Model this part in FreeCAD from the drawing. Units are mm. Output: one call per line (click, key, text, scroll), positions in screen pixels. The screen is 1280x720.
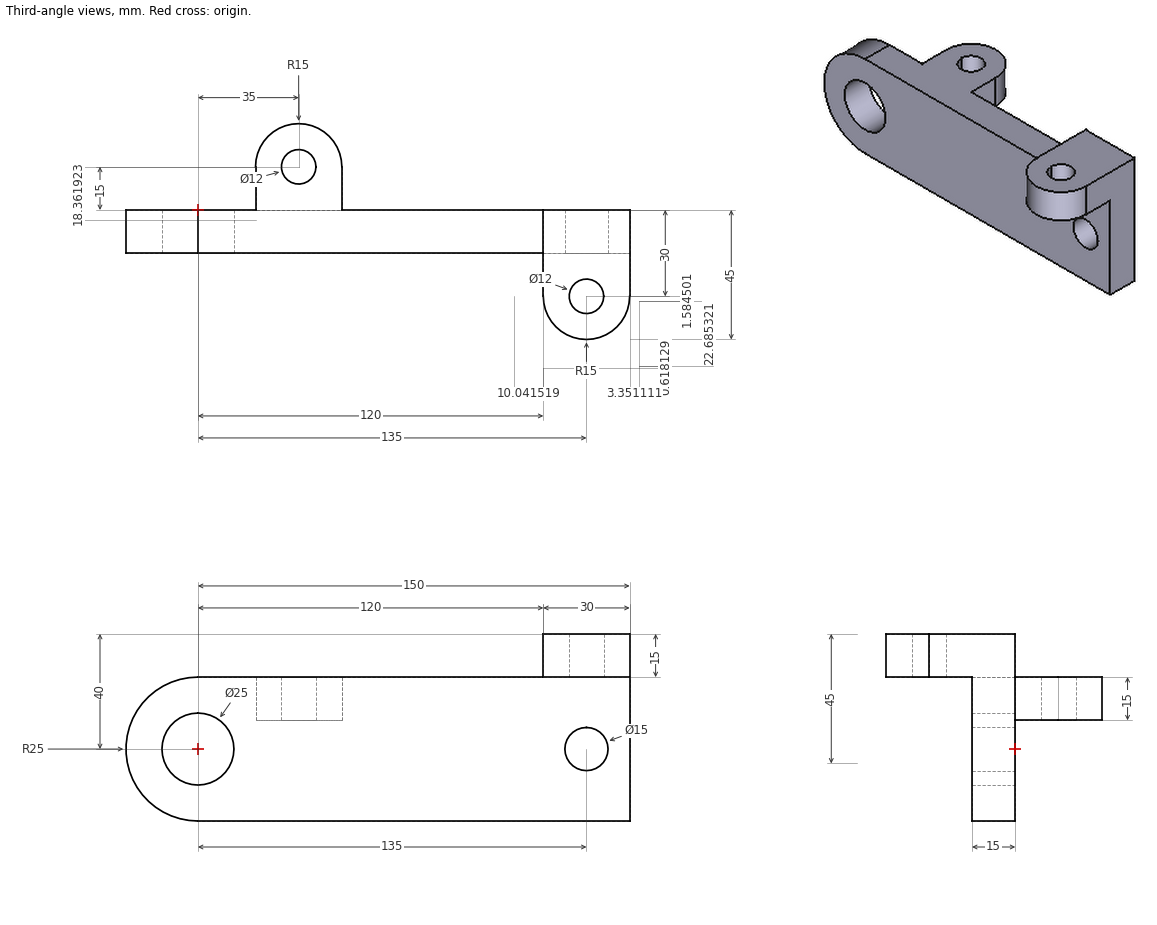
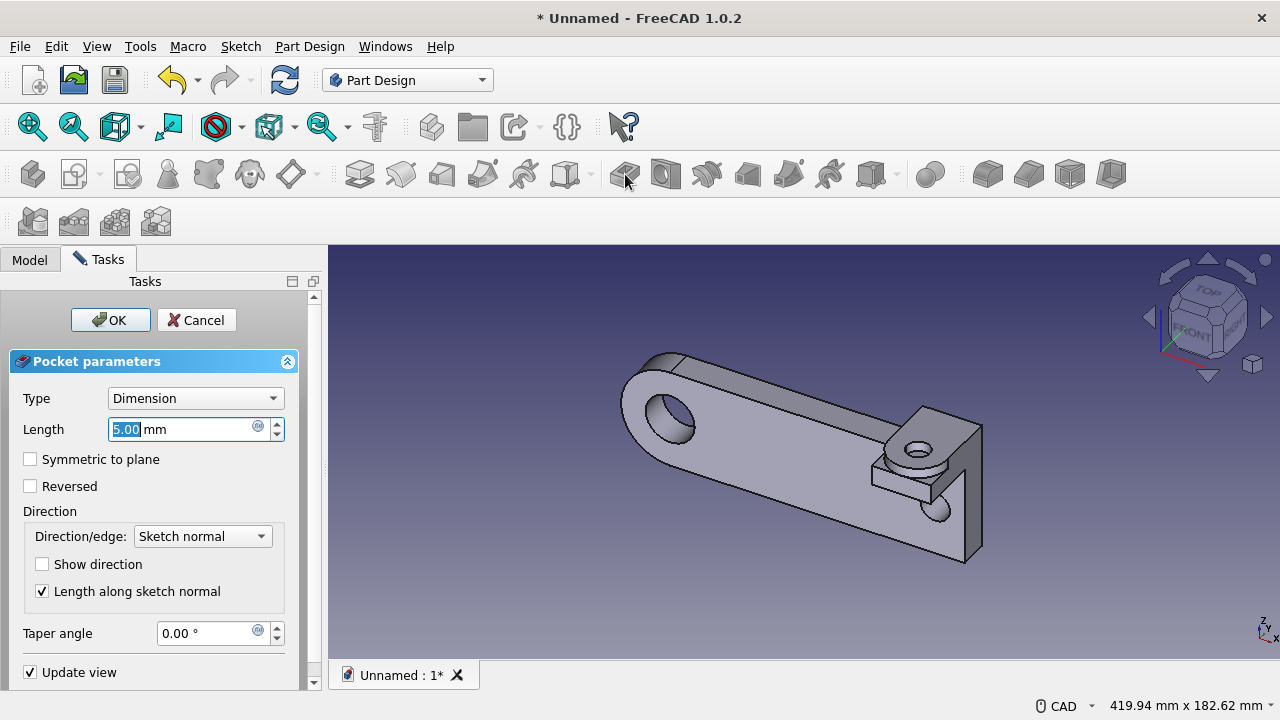
text(45)
key(Tab)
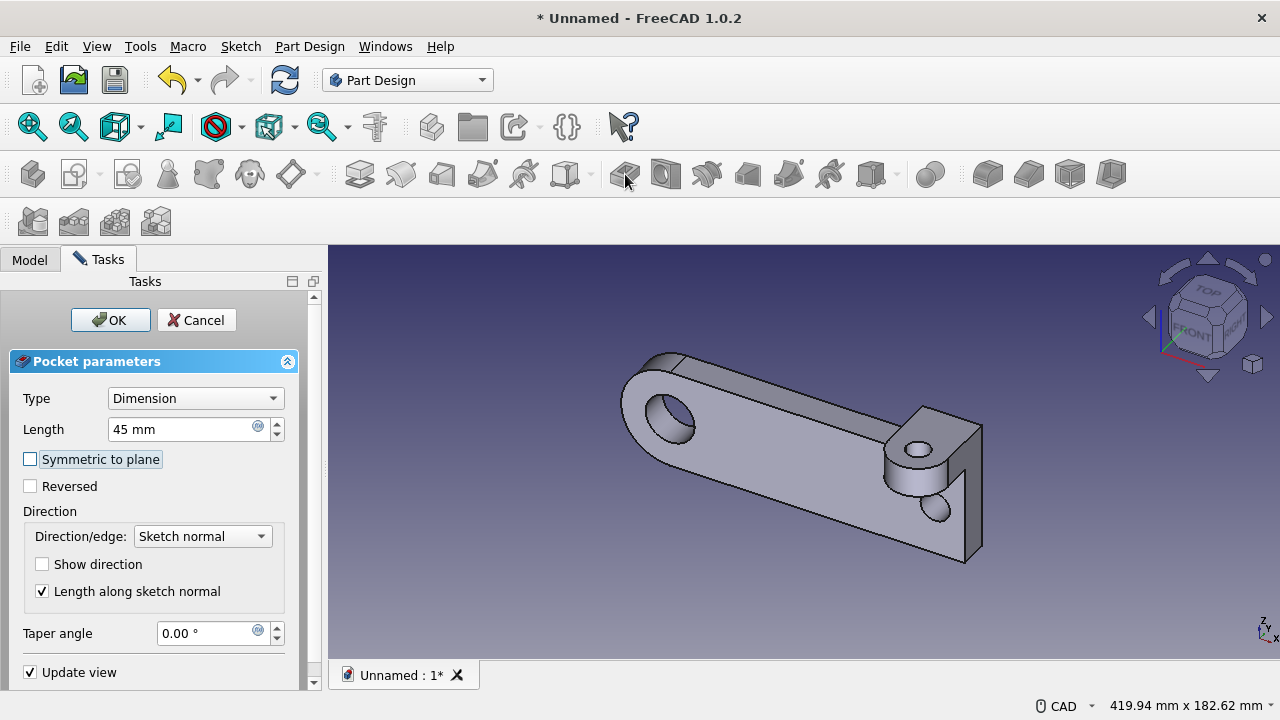
click(111, 320)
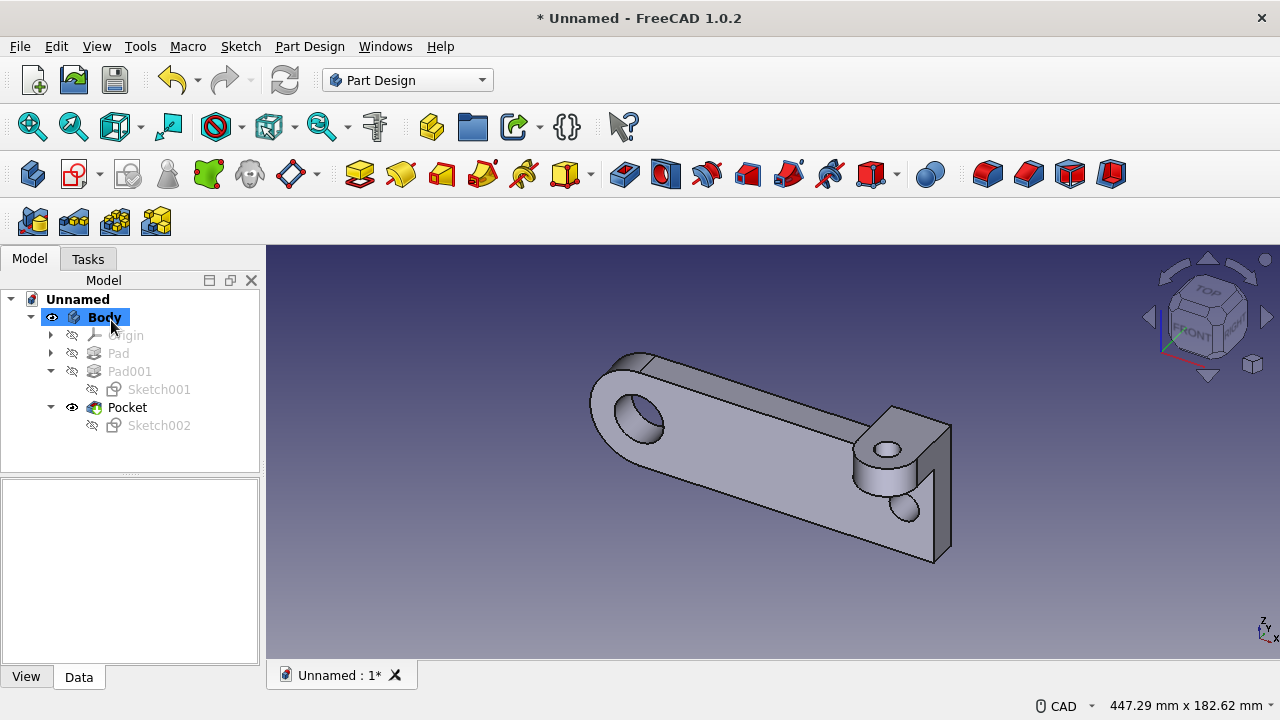
click(833, 425)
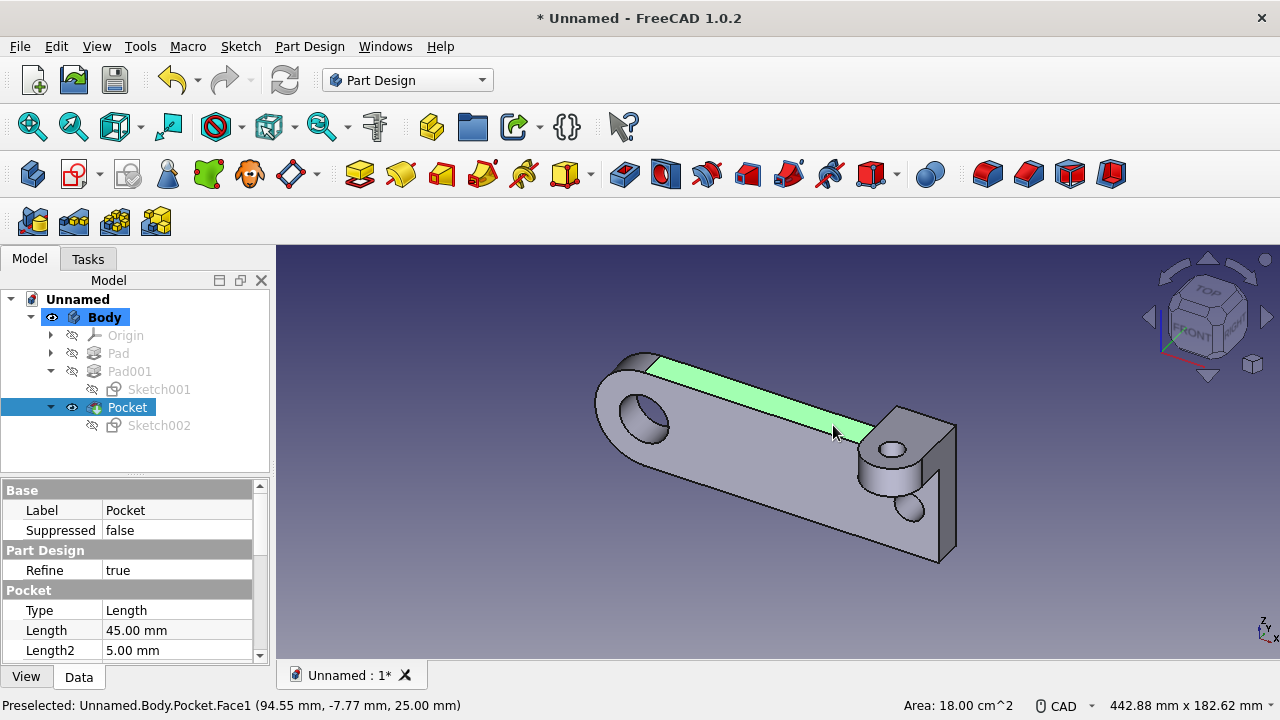
click(74, 174)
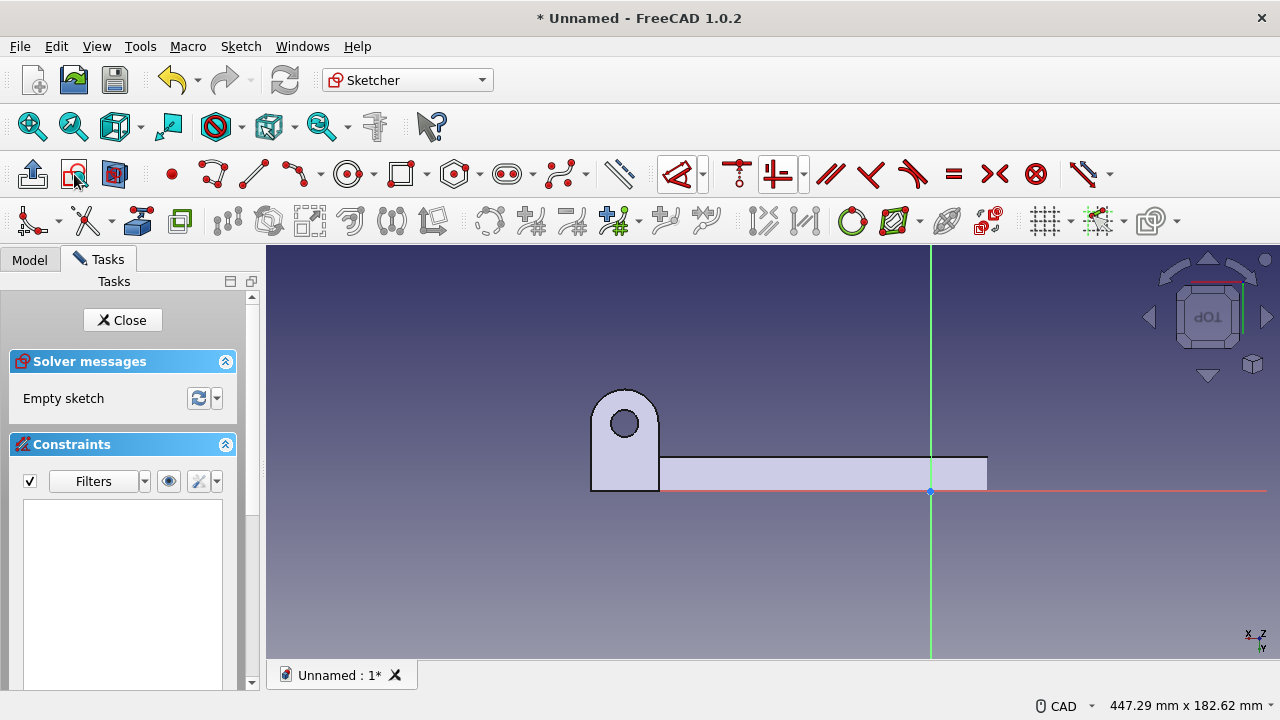
click(115, 174)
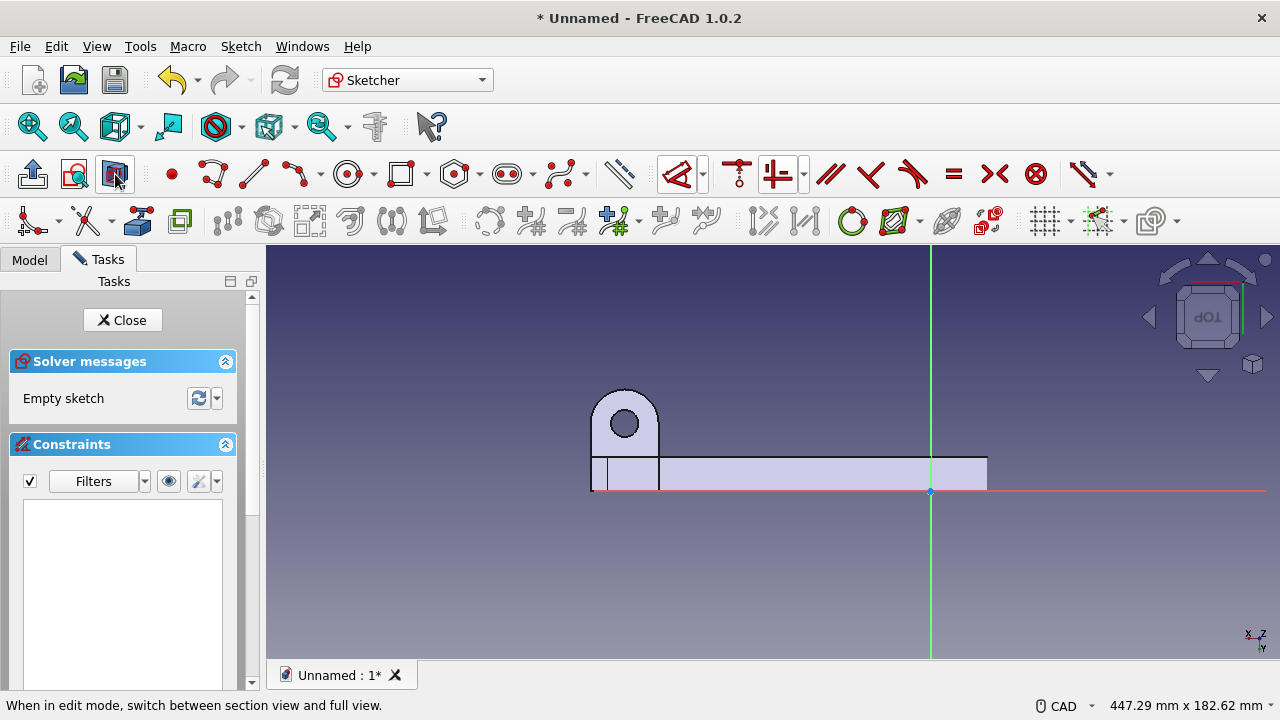
scroll(947, 552, up, 6)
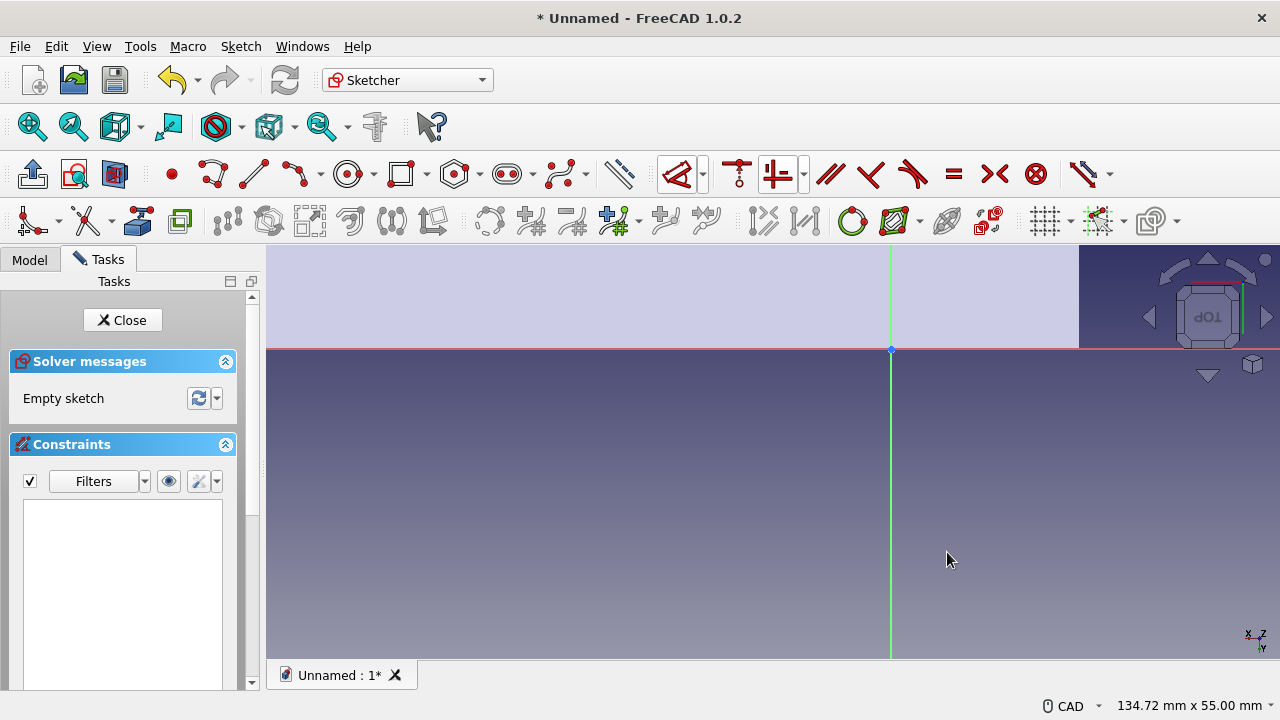
click(213, 174)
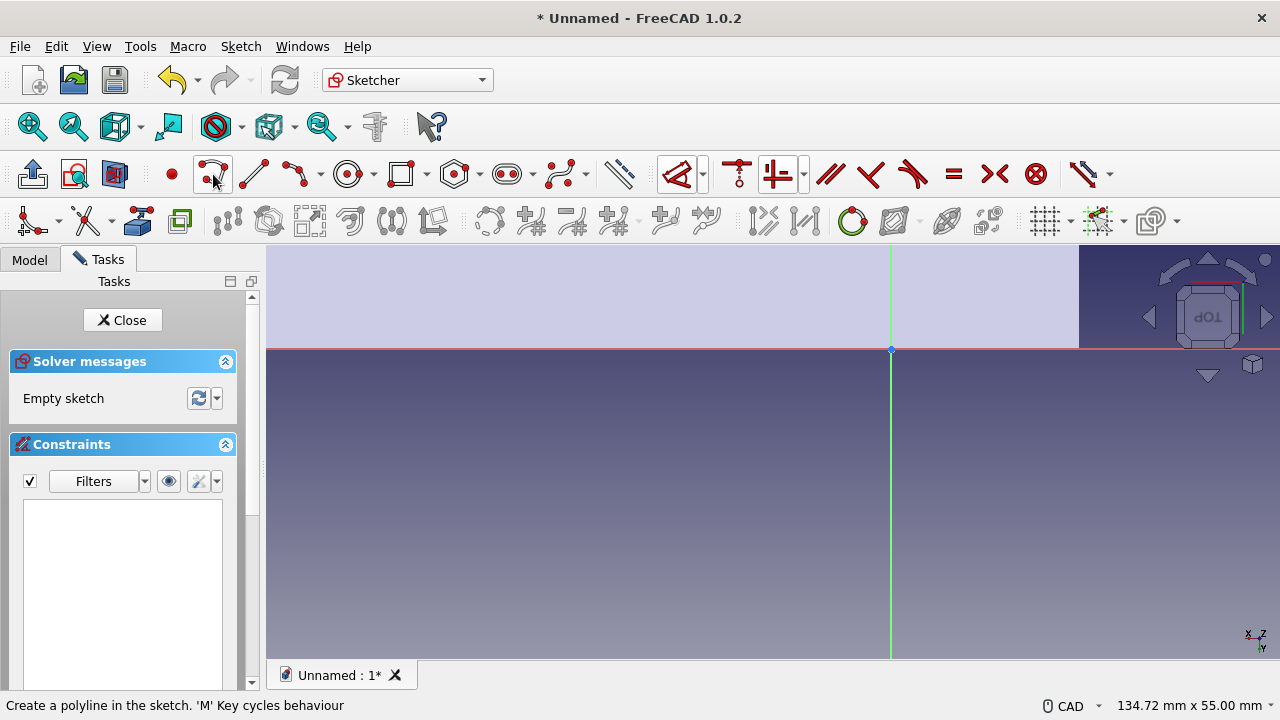
click(741, 462)
click(741, 324)
click(515, 324)
click(515, 462)
right_click(515, 462)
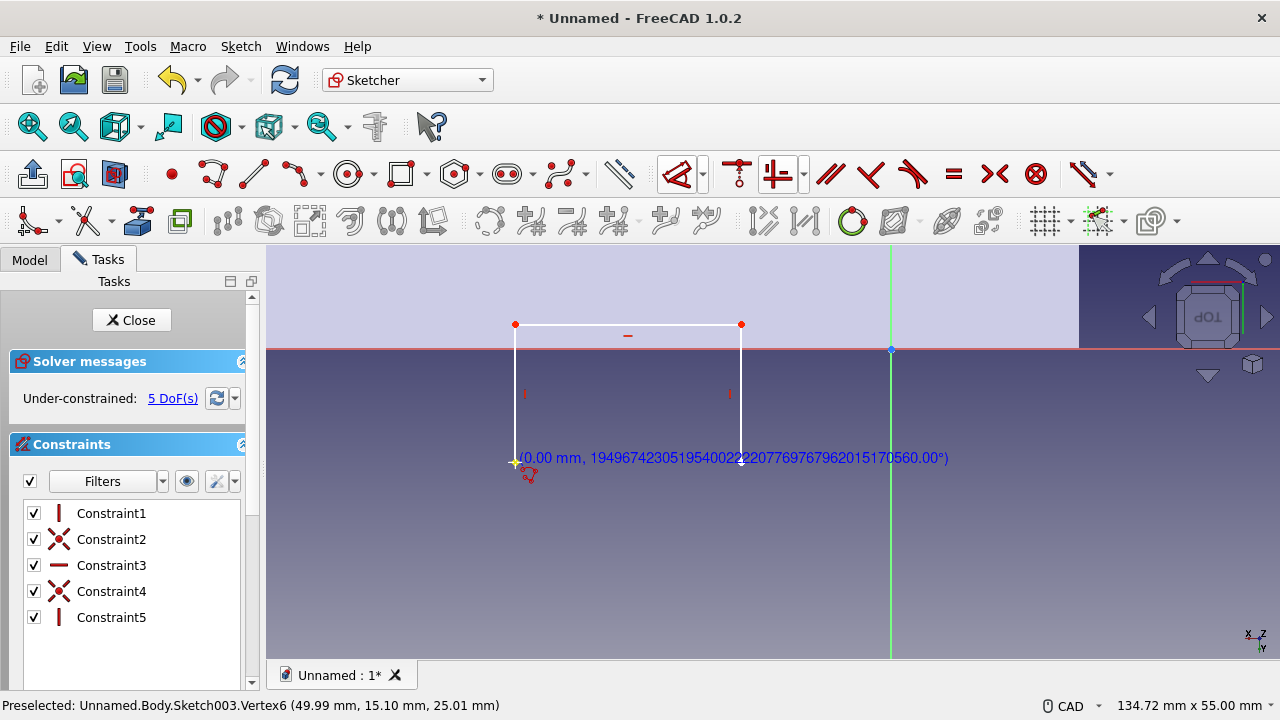
click(294, 174)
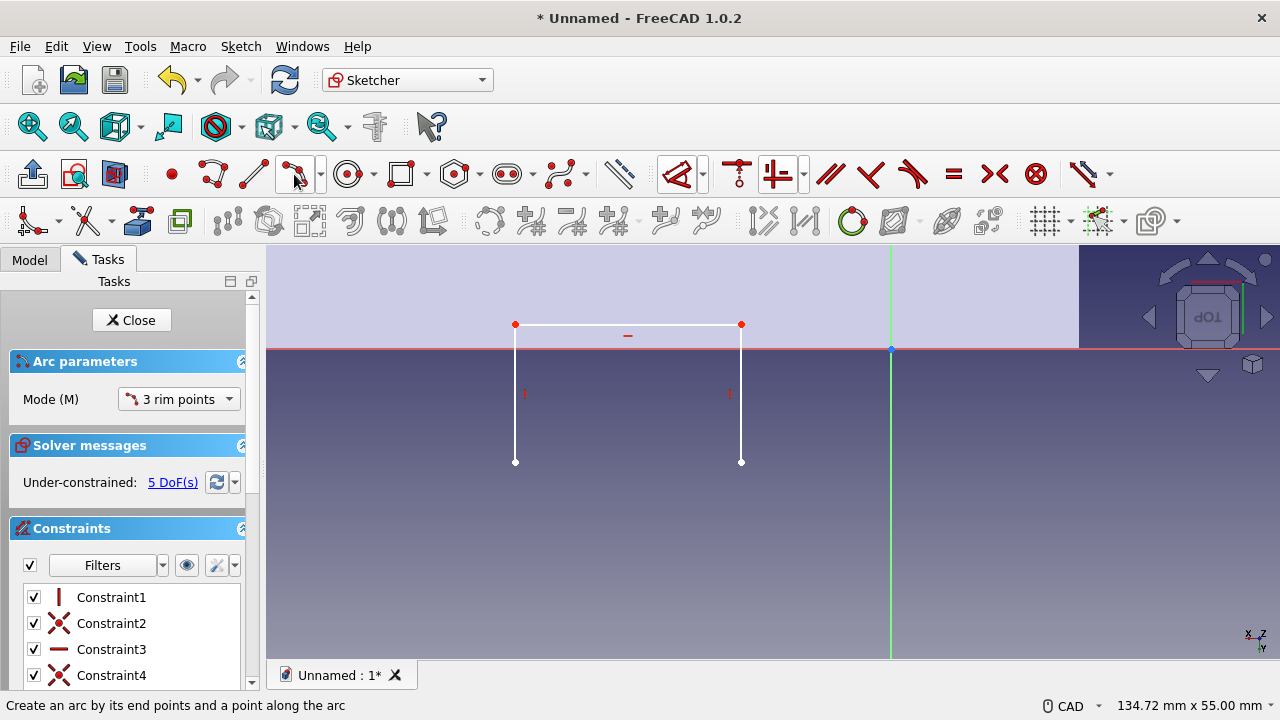
click(515, 463)
click(741, 463)
click(628, 575)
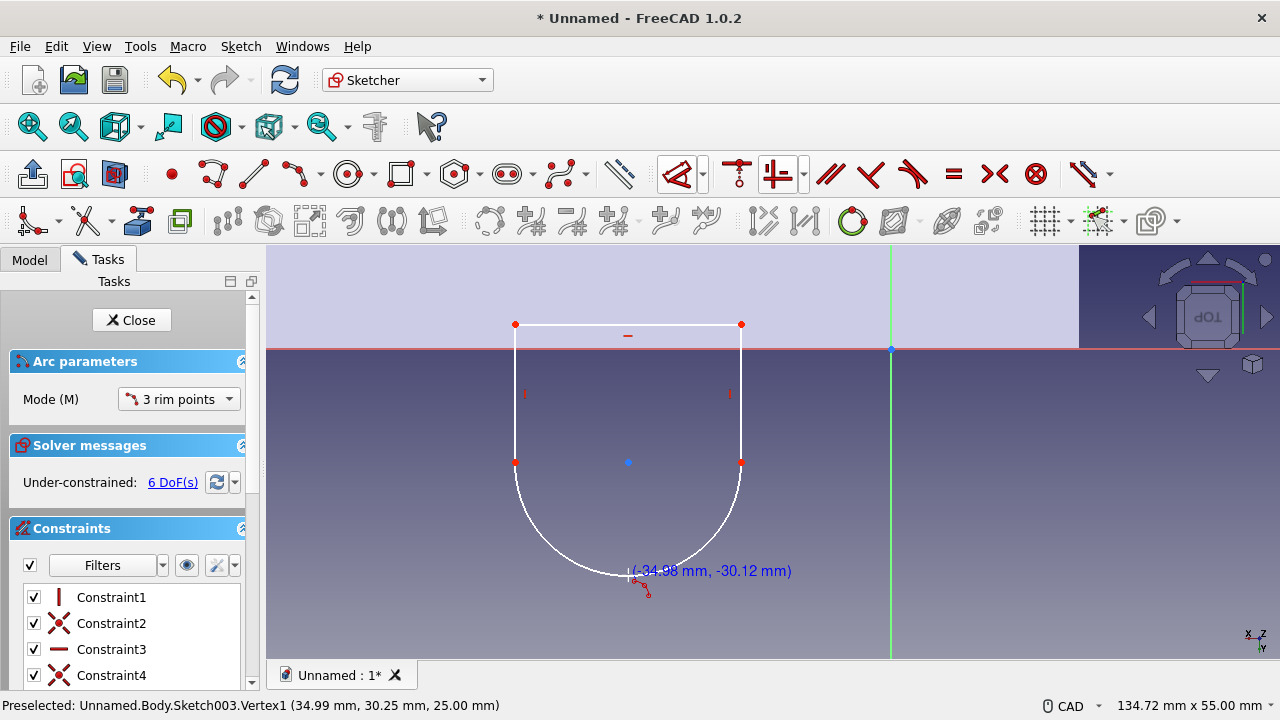
click(348, 174)